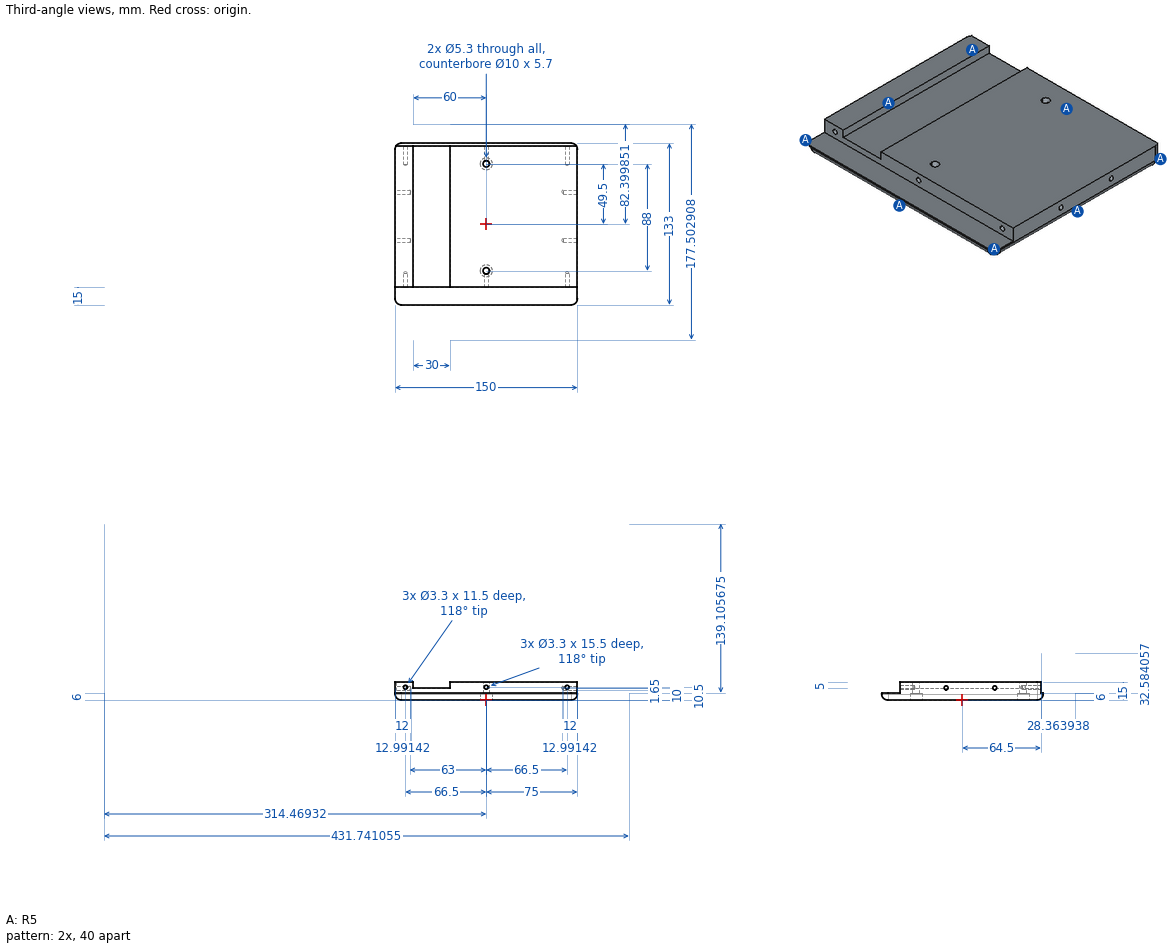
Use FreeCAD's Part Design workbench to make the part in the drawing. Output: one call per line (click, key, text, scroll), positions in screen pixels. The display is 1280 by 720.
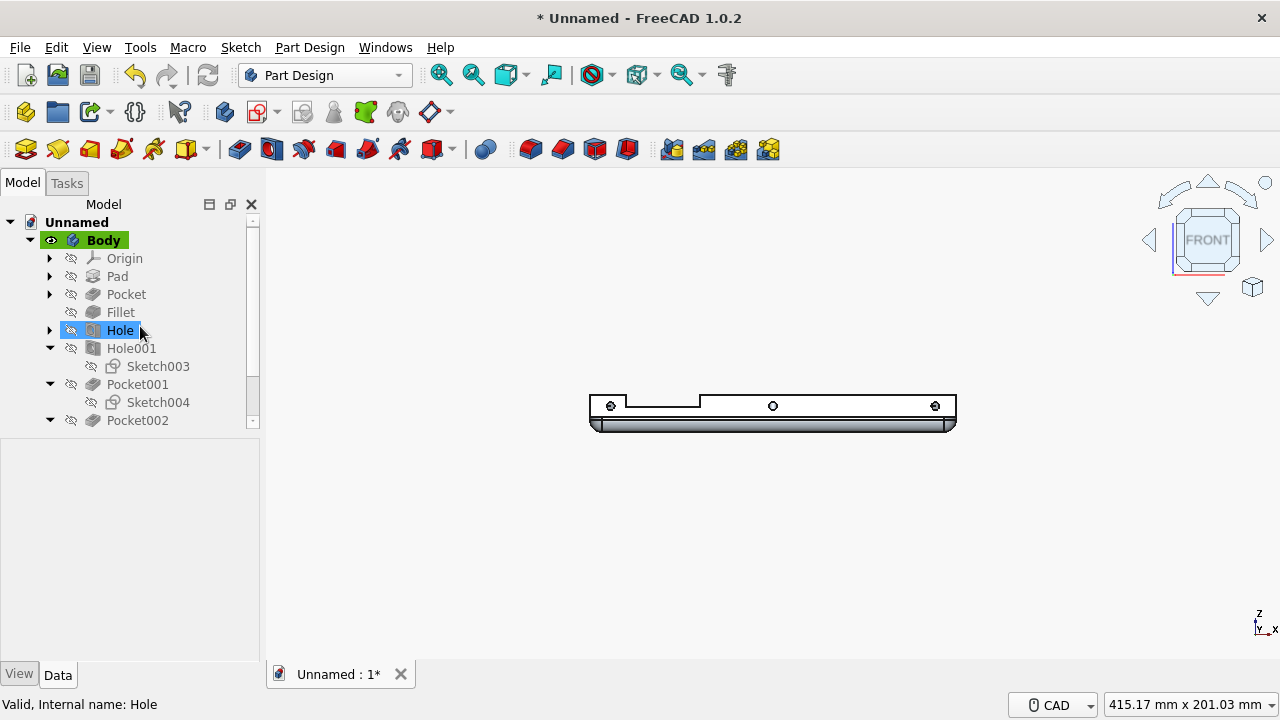
click(50, 258)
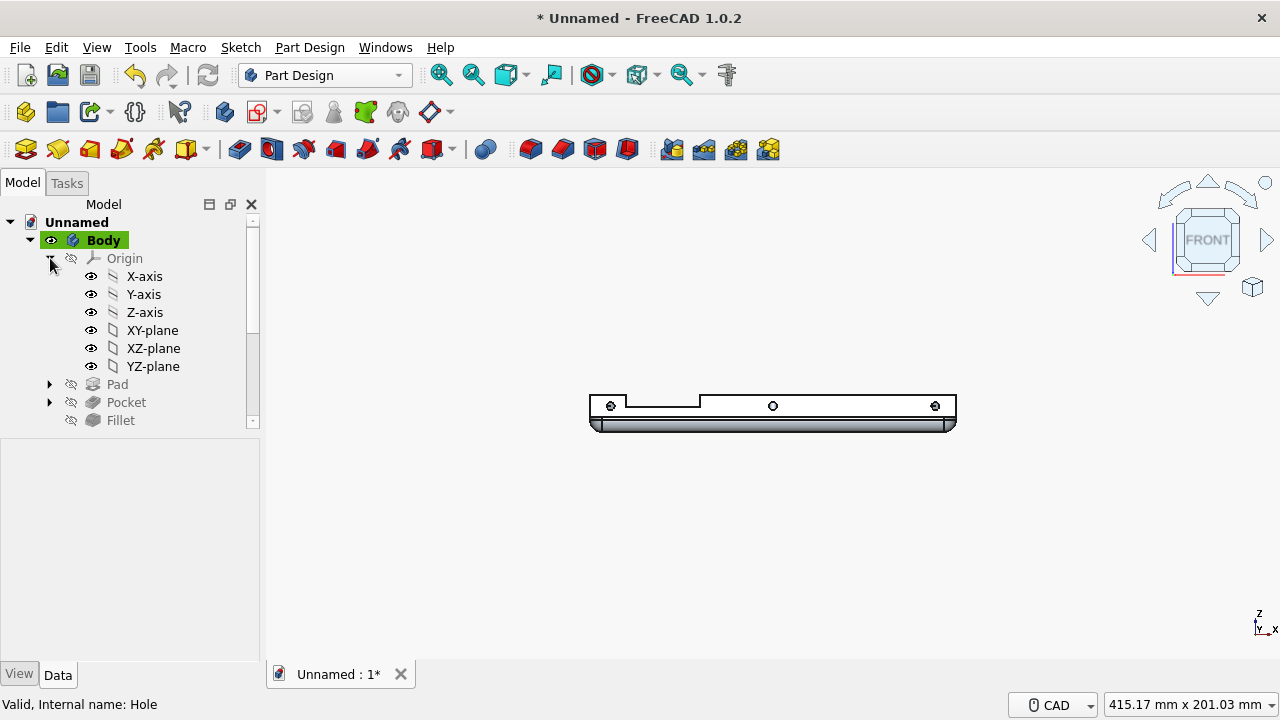
click(136, 348)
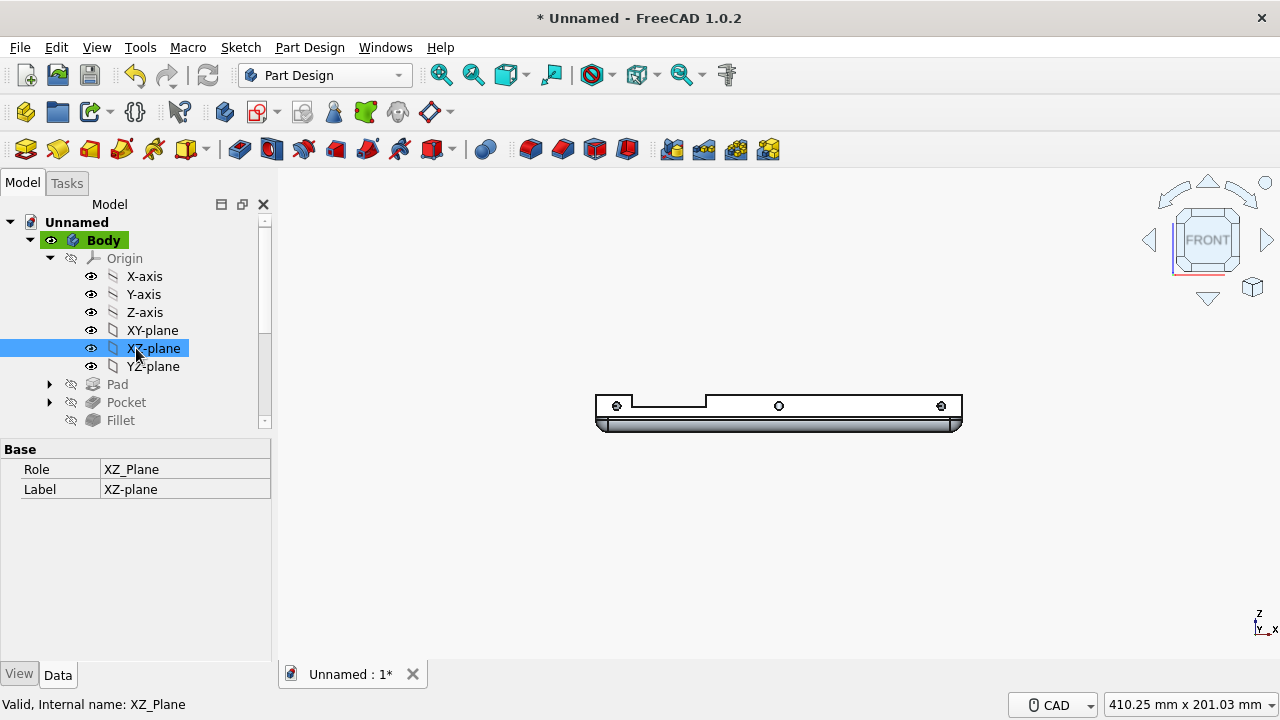
click(430, 112)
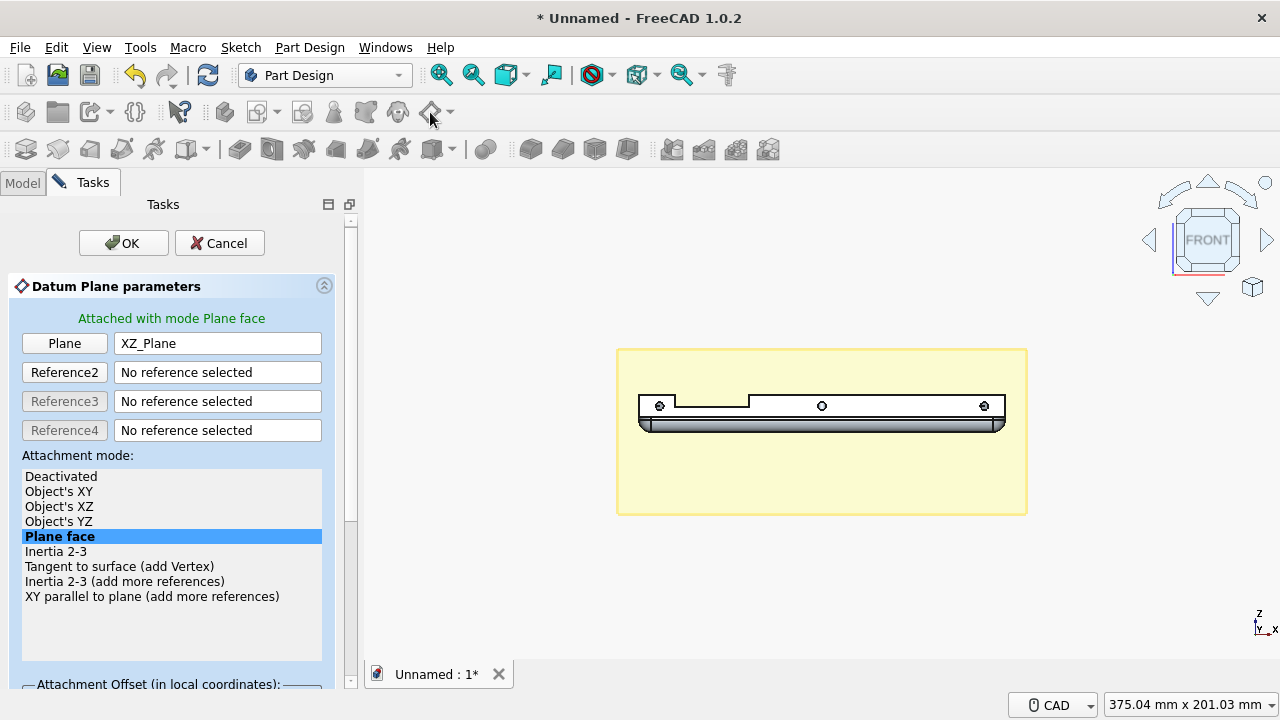
scroll(351, 451, down, 3)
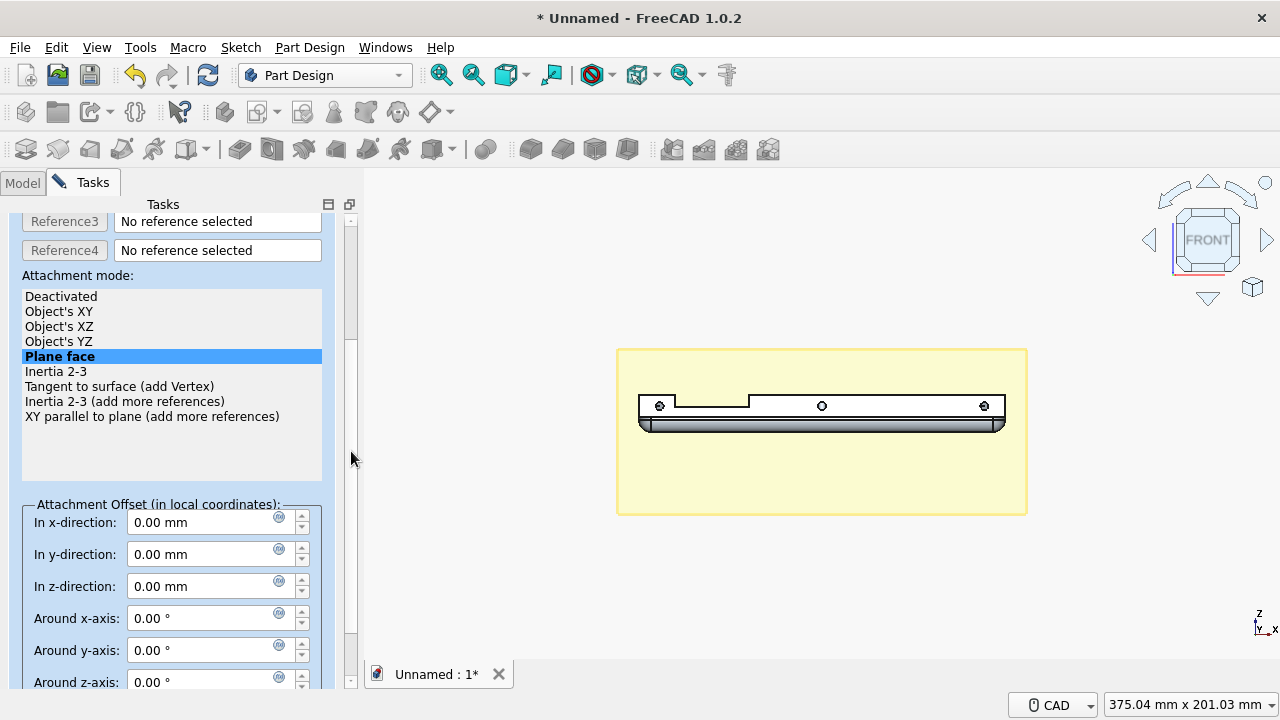
triple_click(210, 586)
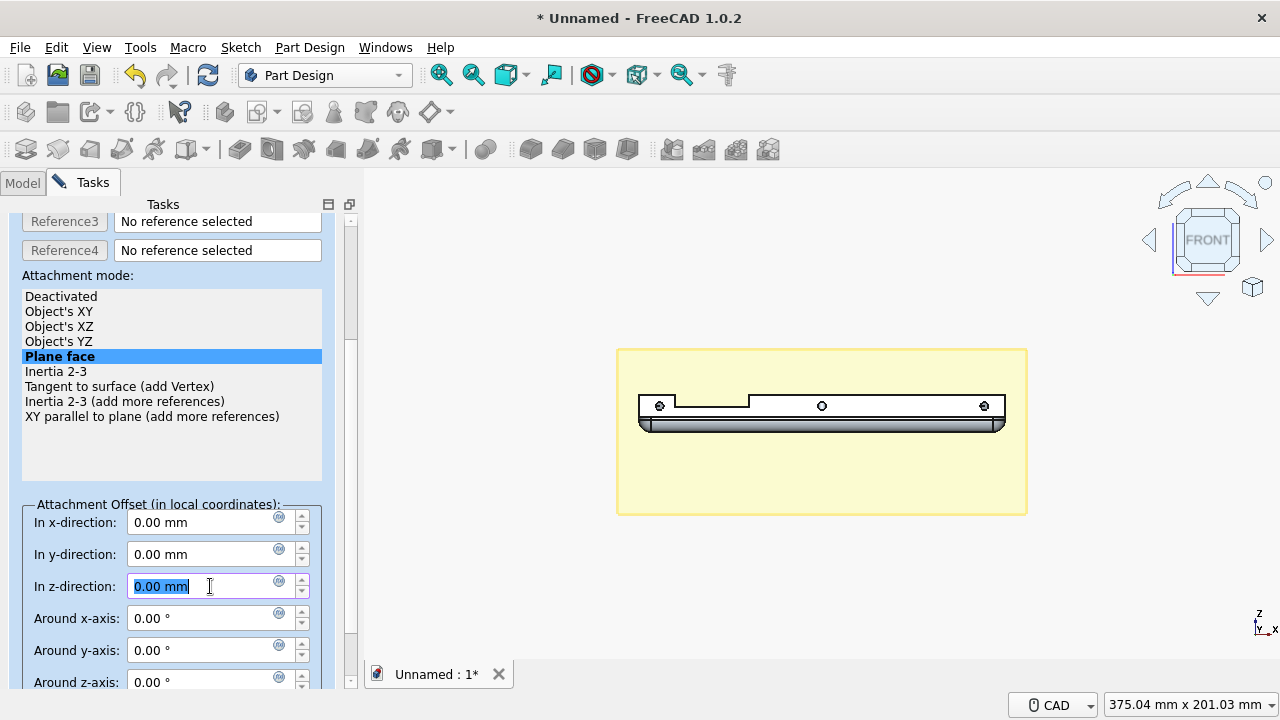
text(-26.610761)
key(Tab)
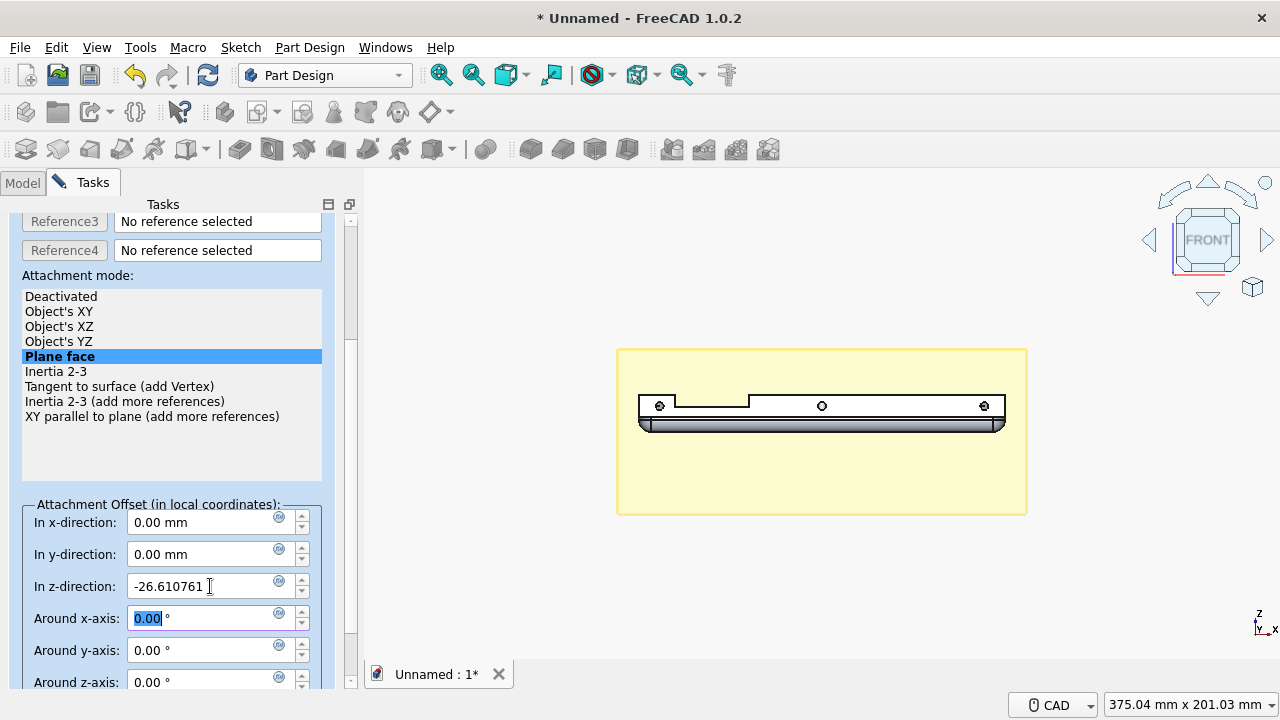
scroll(351, 451, up, 4)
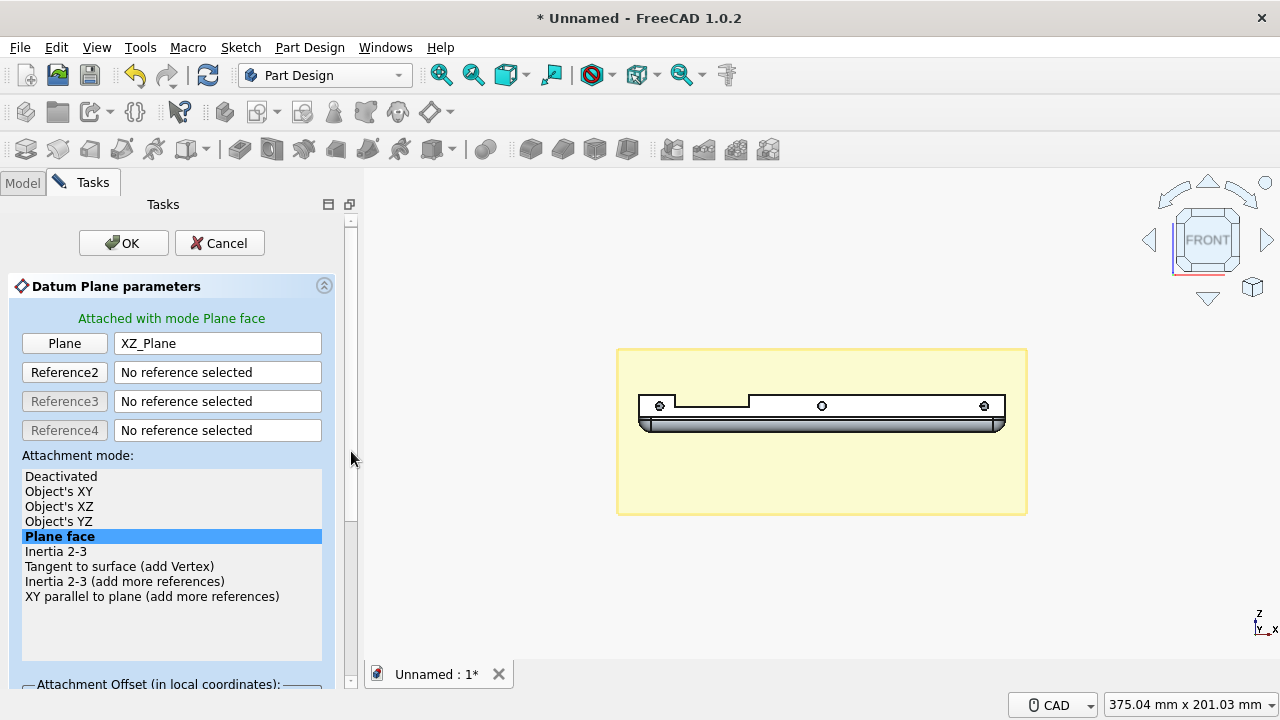
click(124, 243)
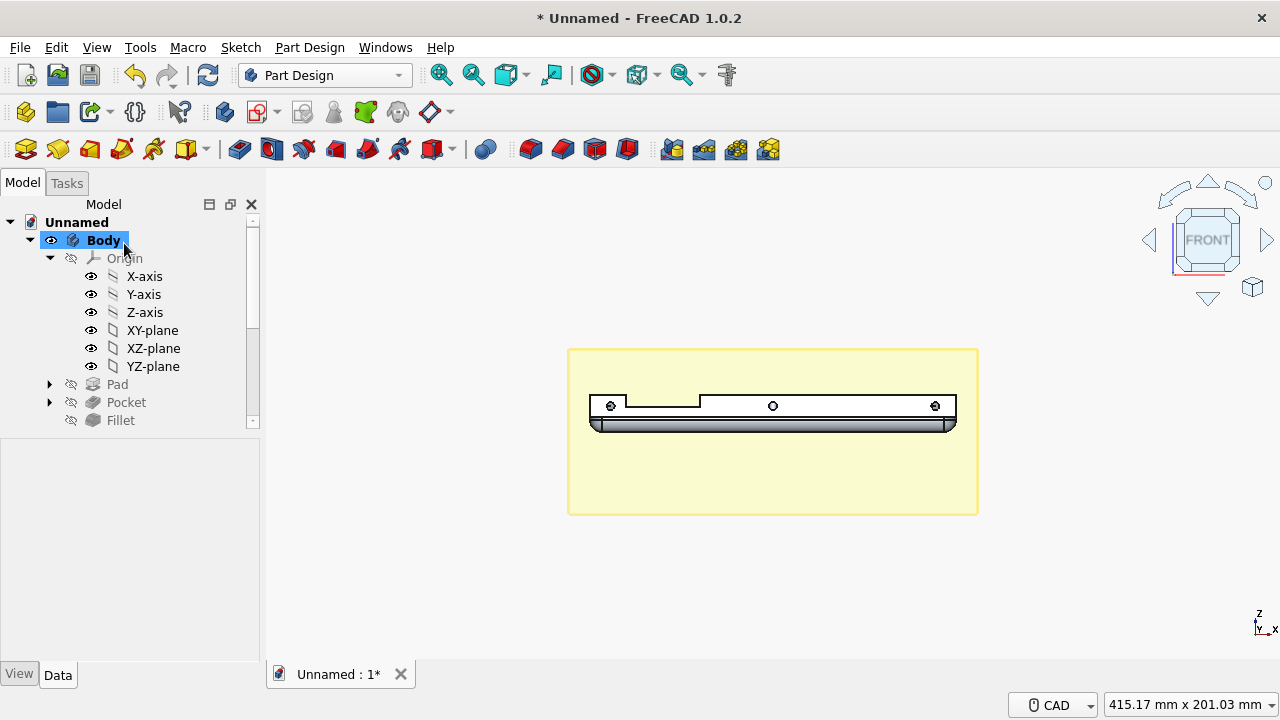
scroll(100, 326, down, 3)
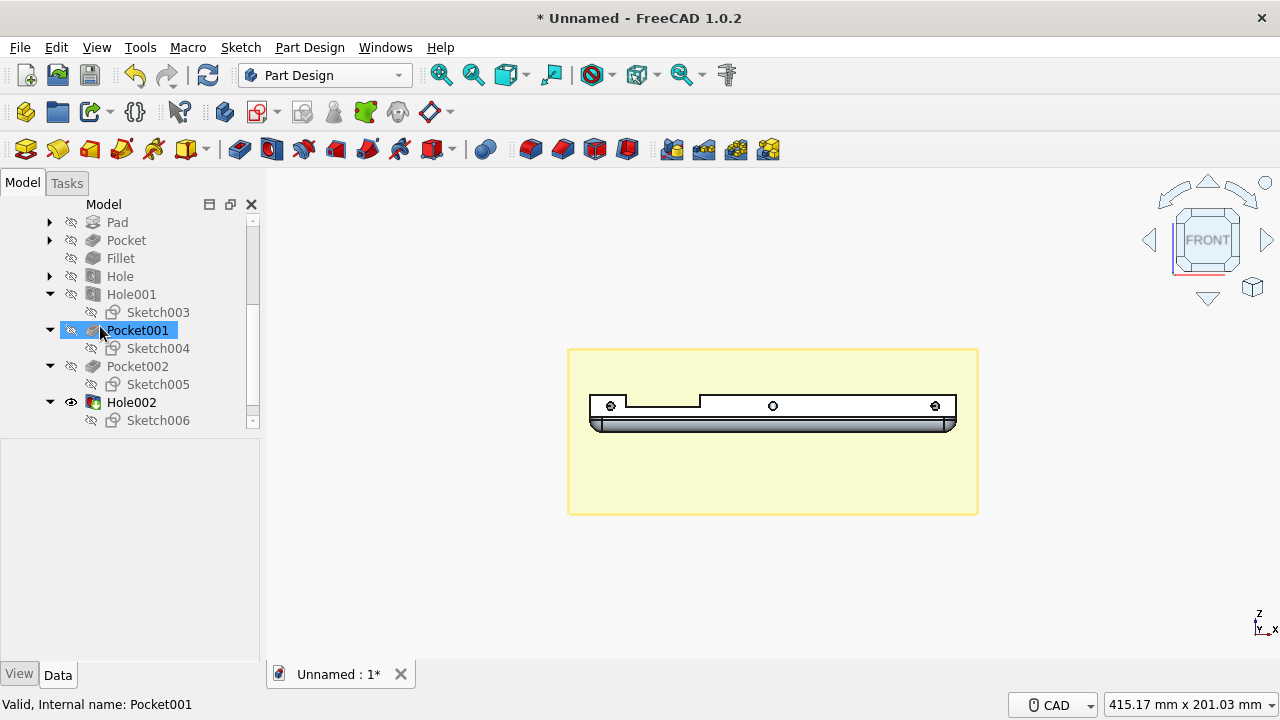
scroll(140, 326, up, 15)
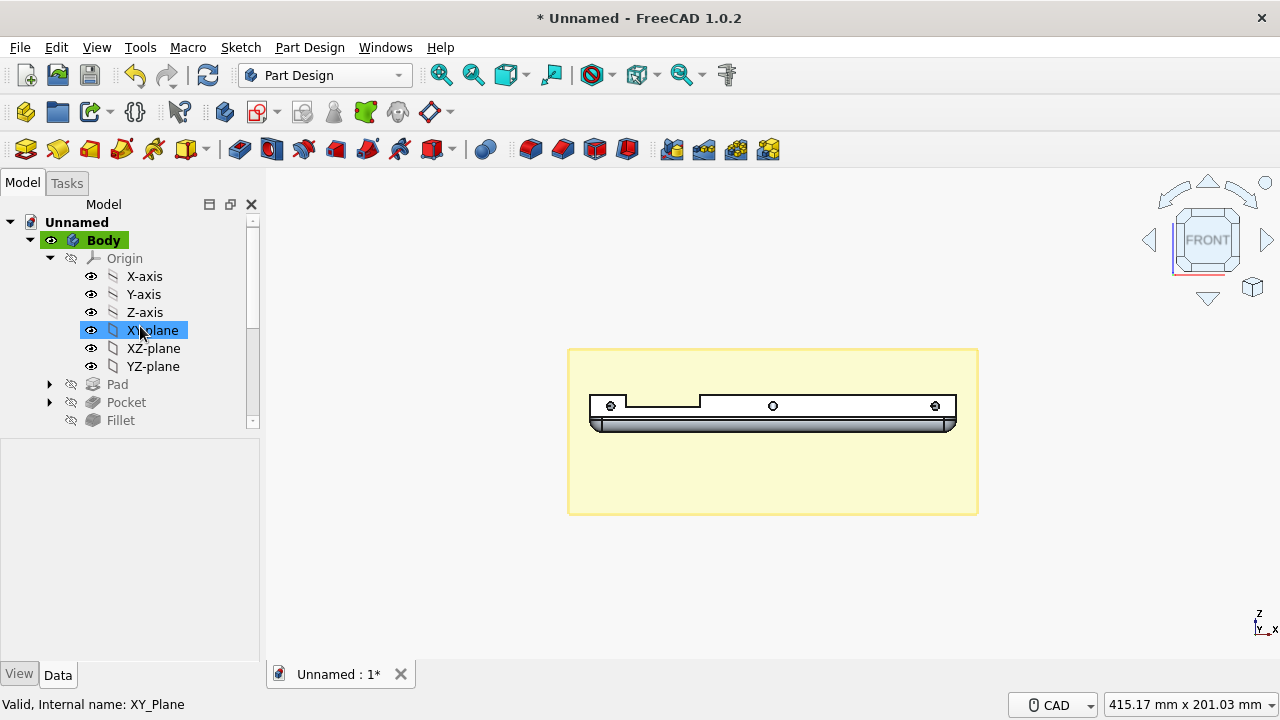
scroll(100, 326, down, 6)